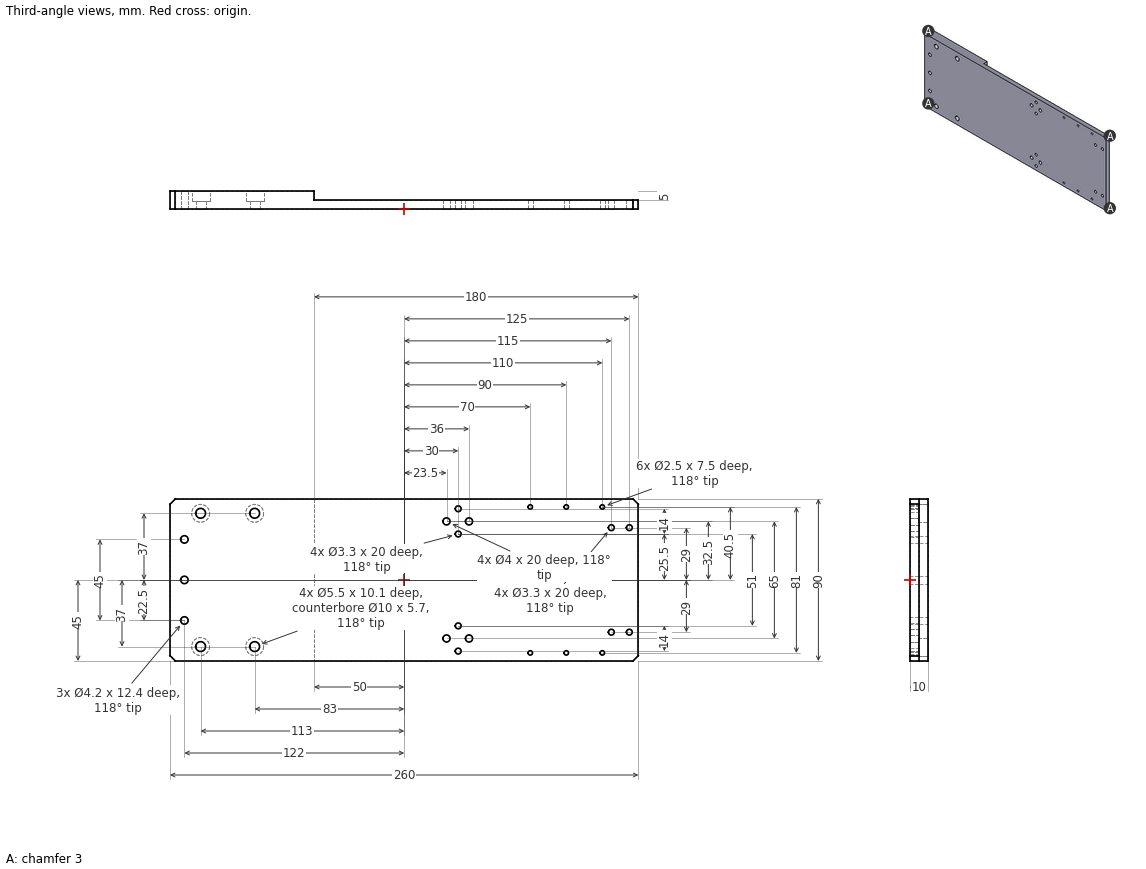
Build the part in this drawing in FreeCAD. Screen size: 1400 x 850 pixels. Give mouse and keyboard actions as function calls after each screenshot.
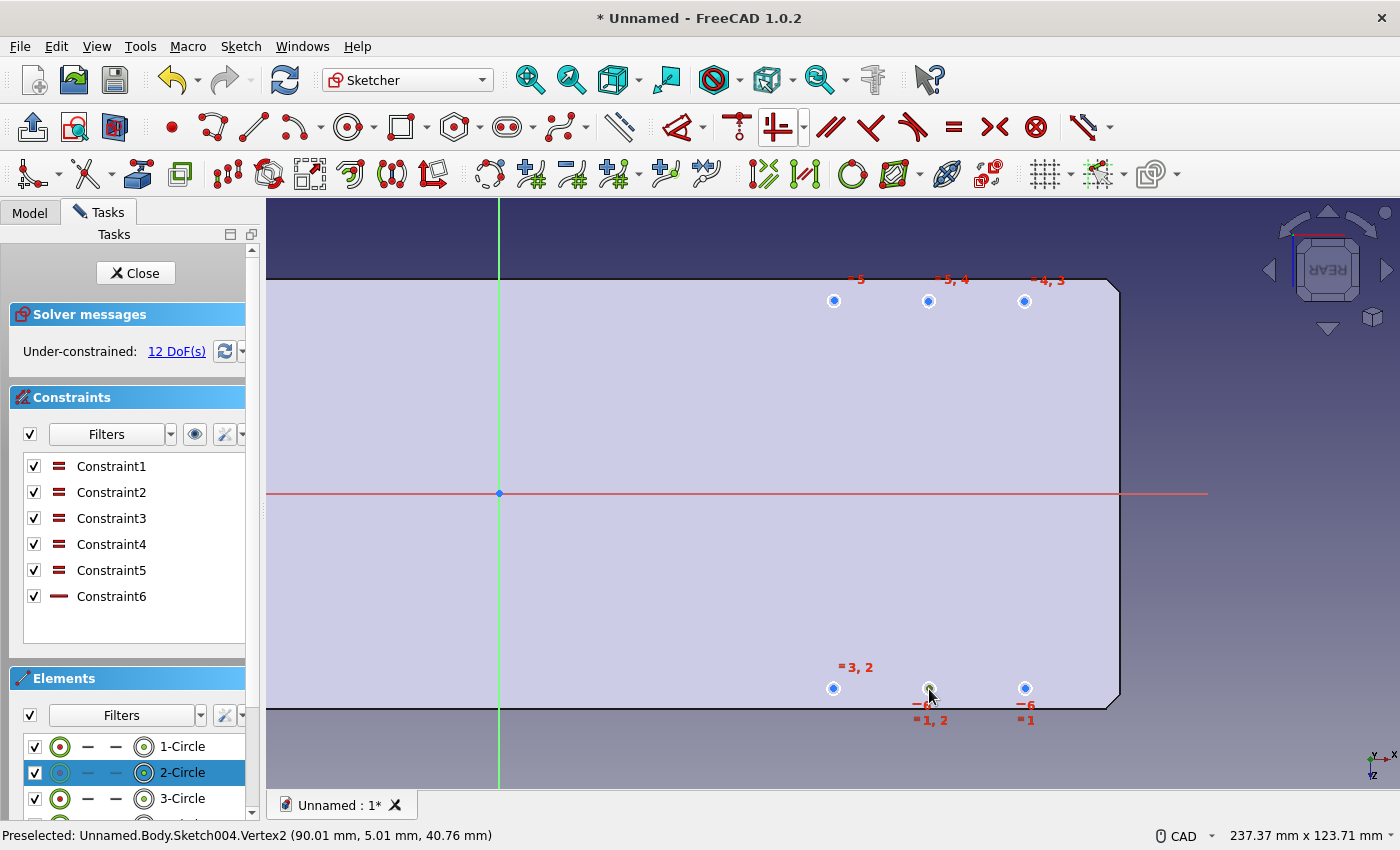
click(834, 689)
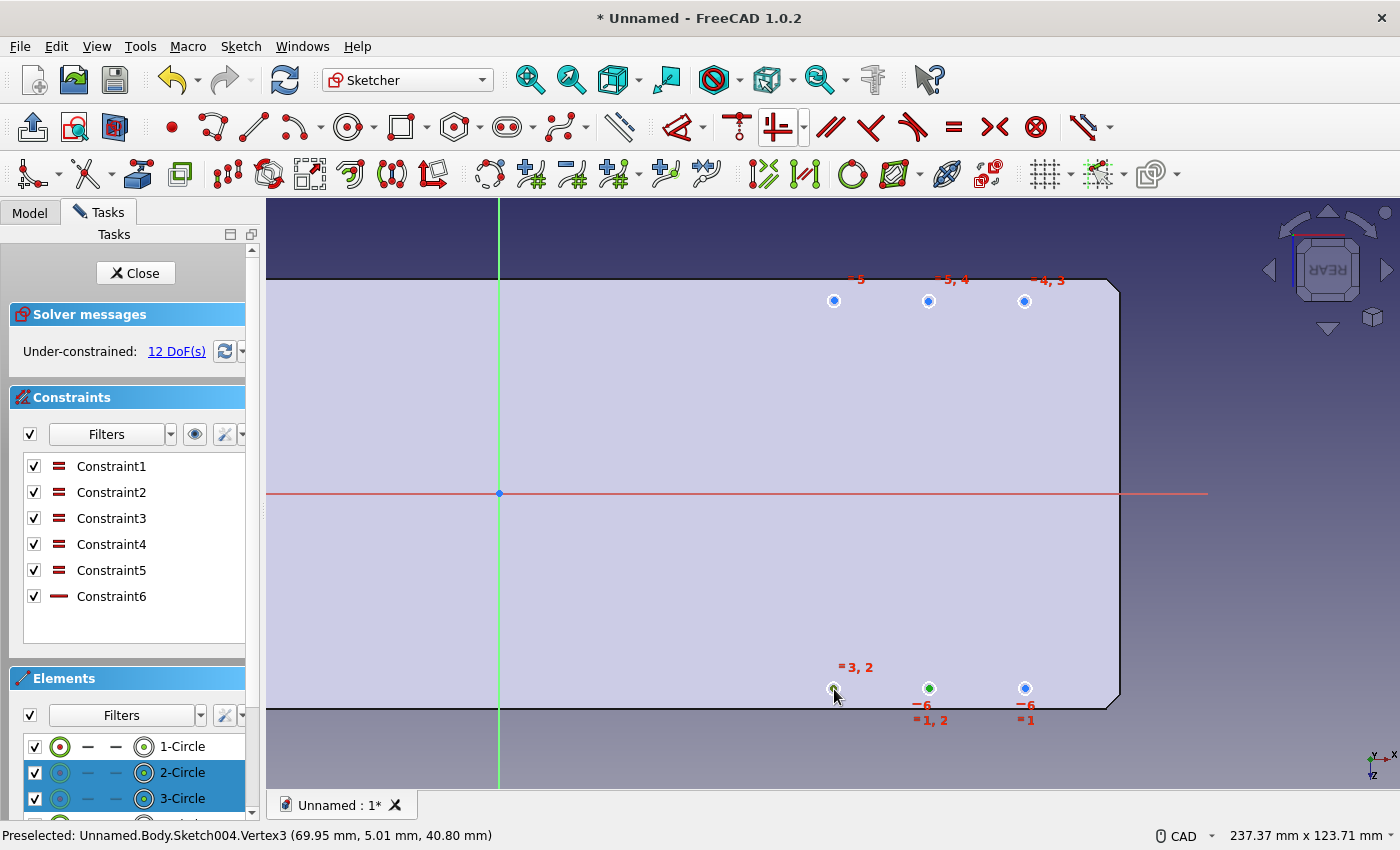
key(h)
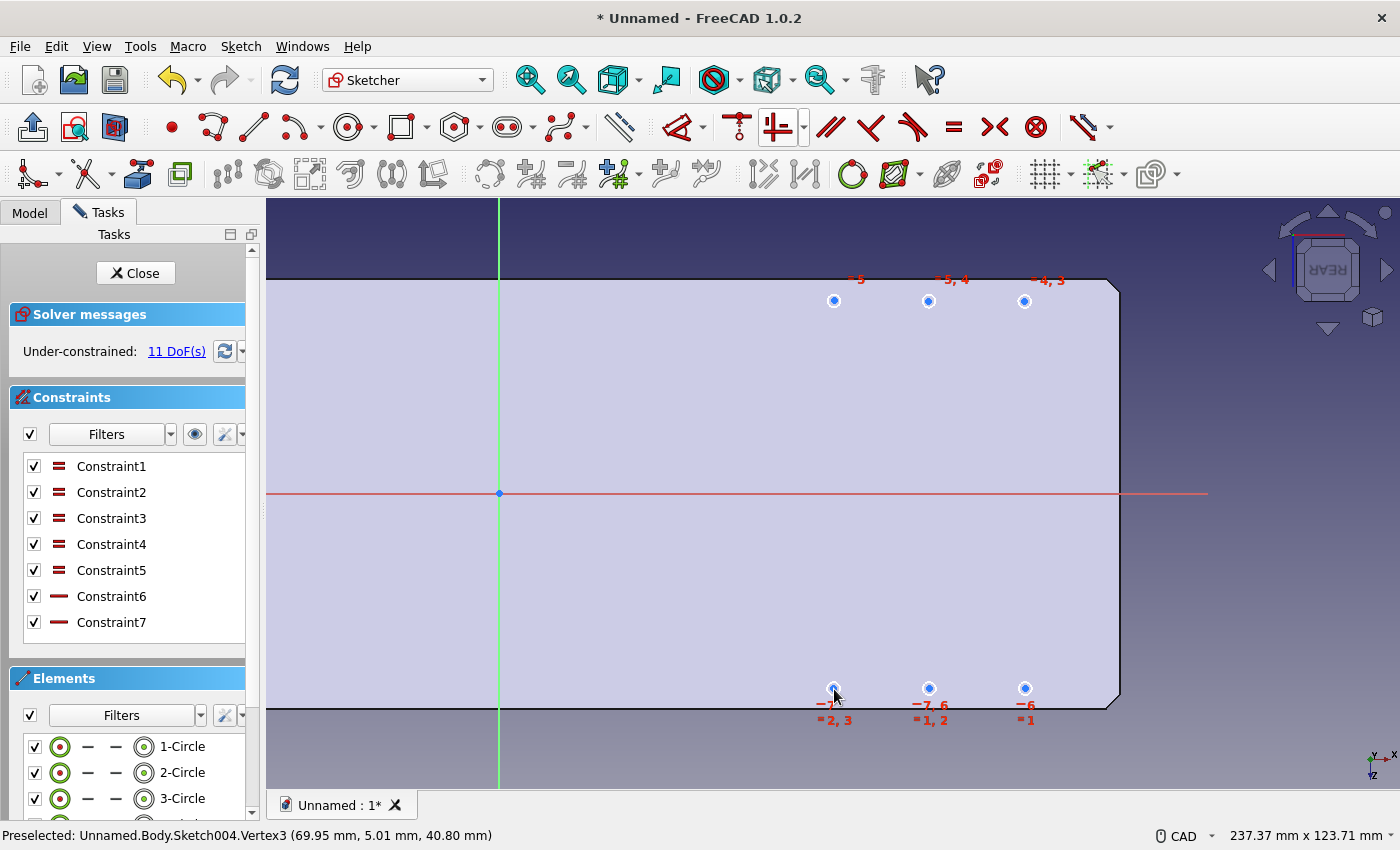
click(1025, 689)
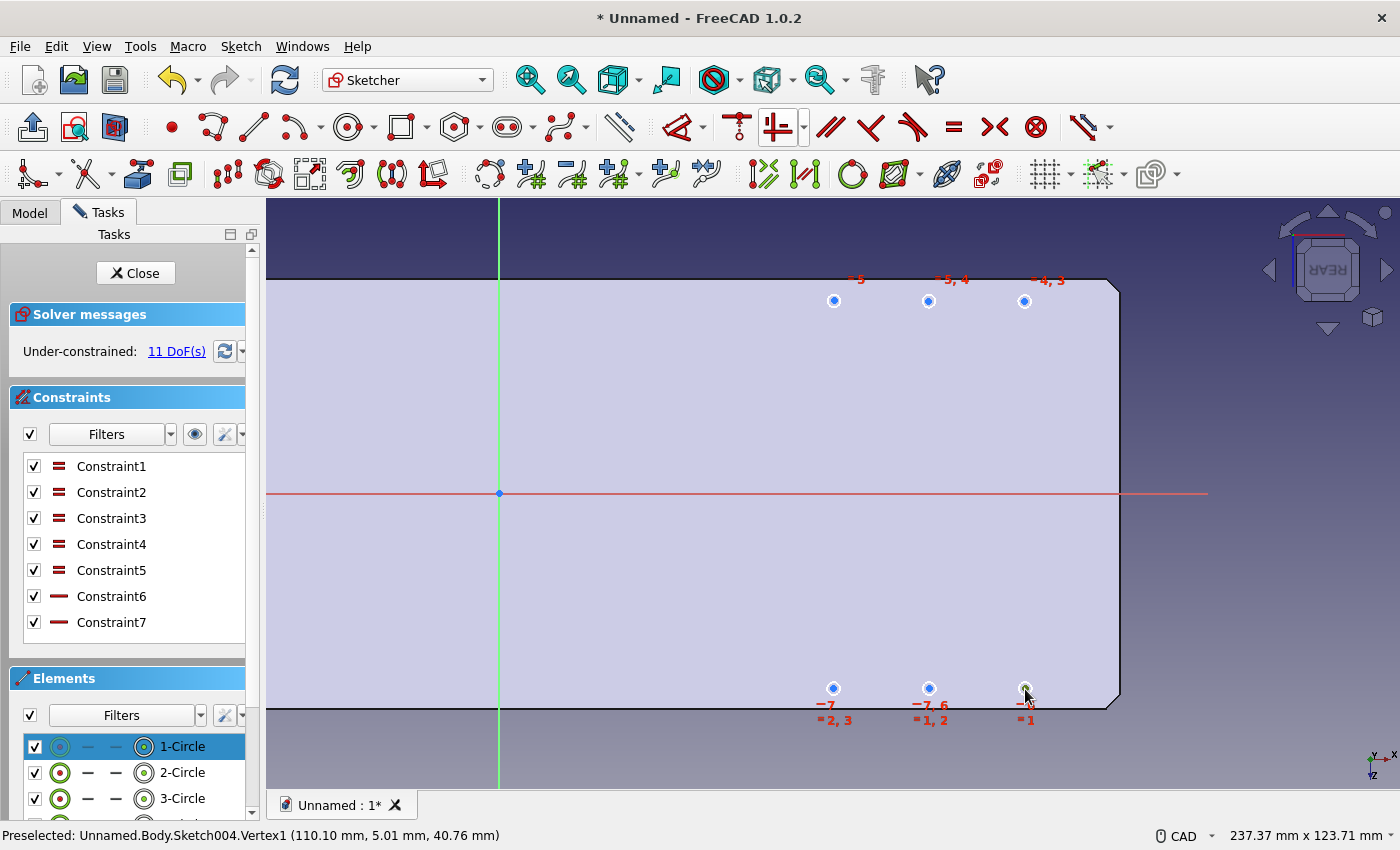
click(1025, 301)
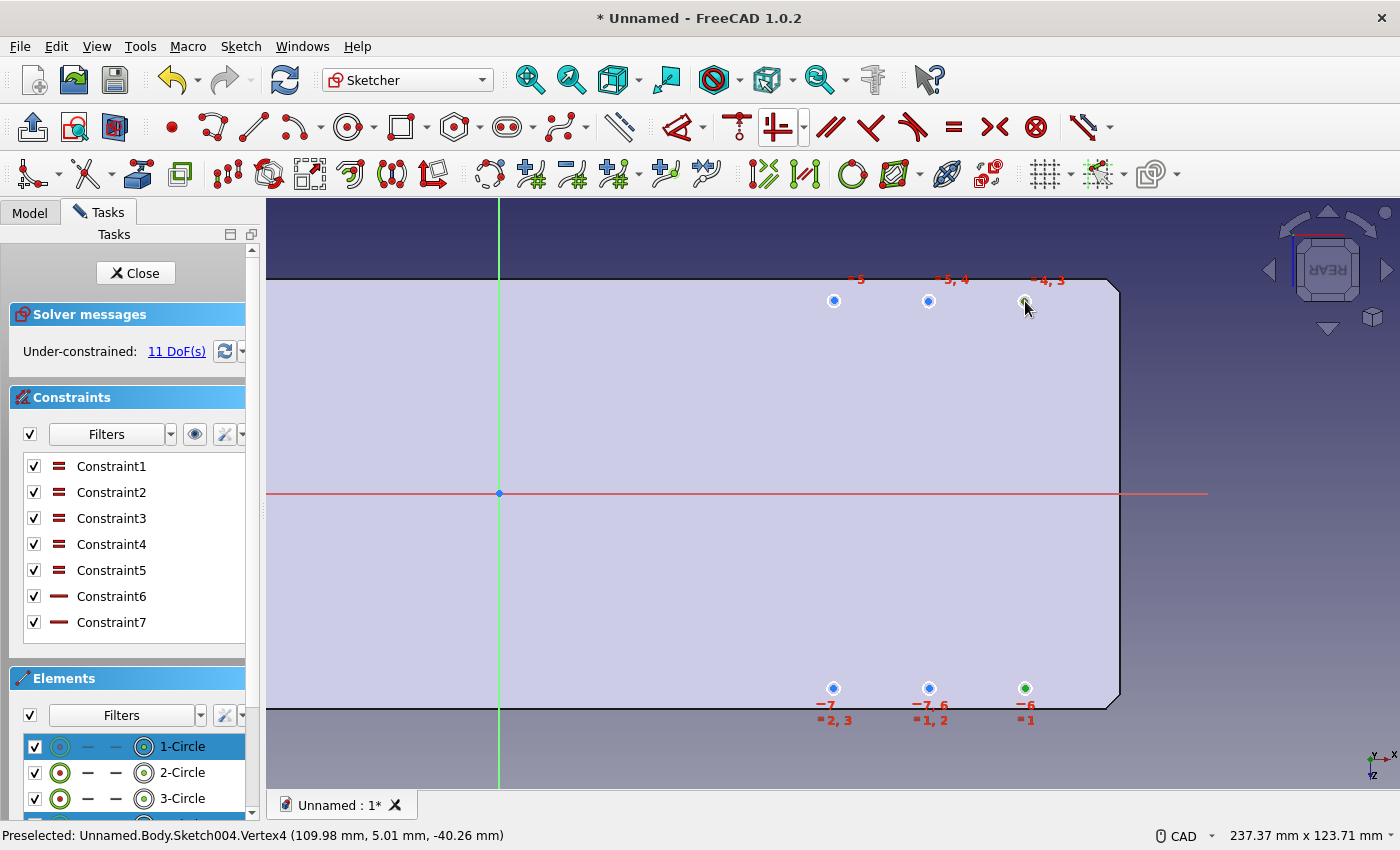
key(v)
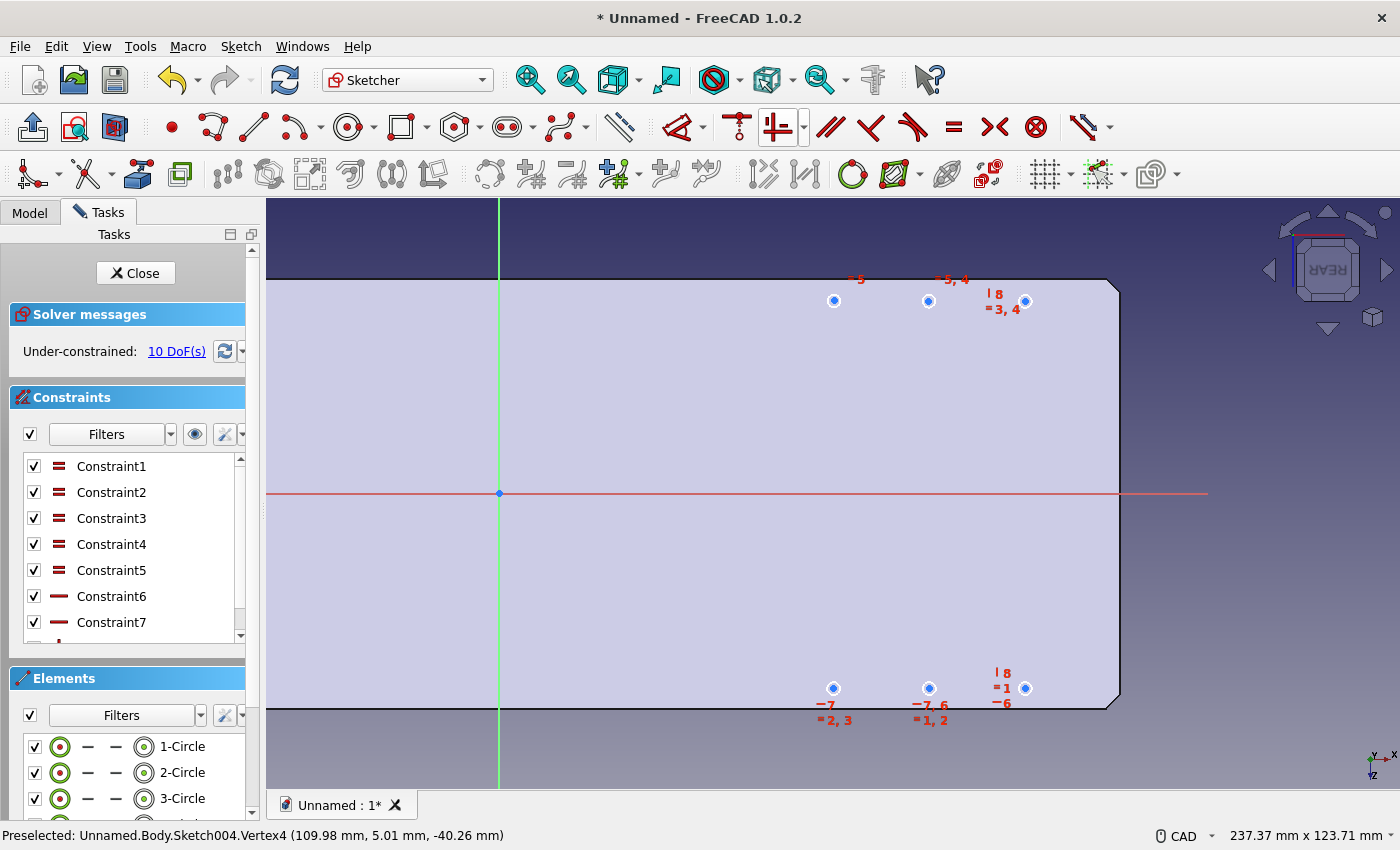
click(929, 689)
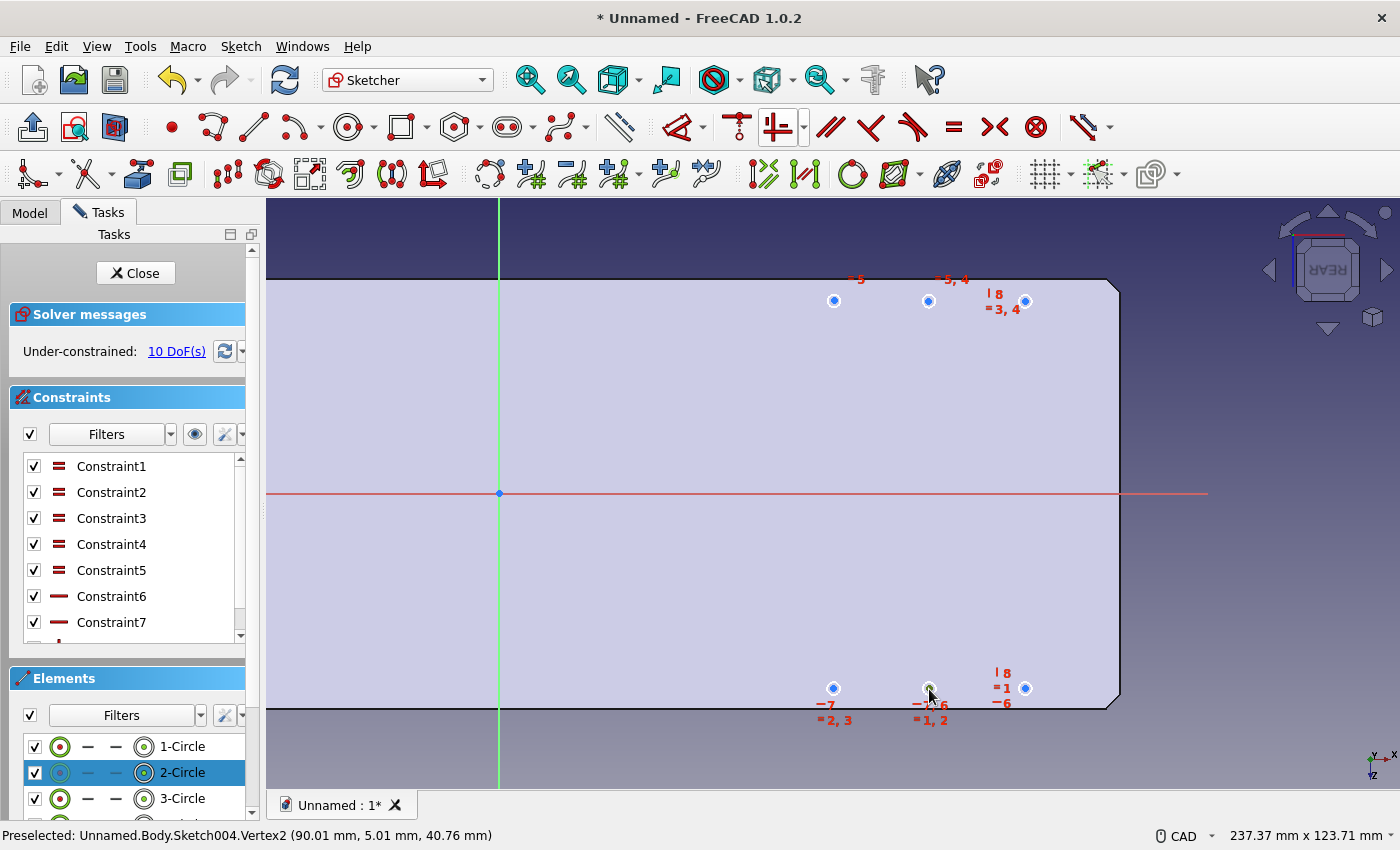
click(929, 301)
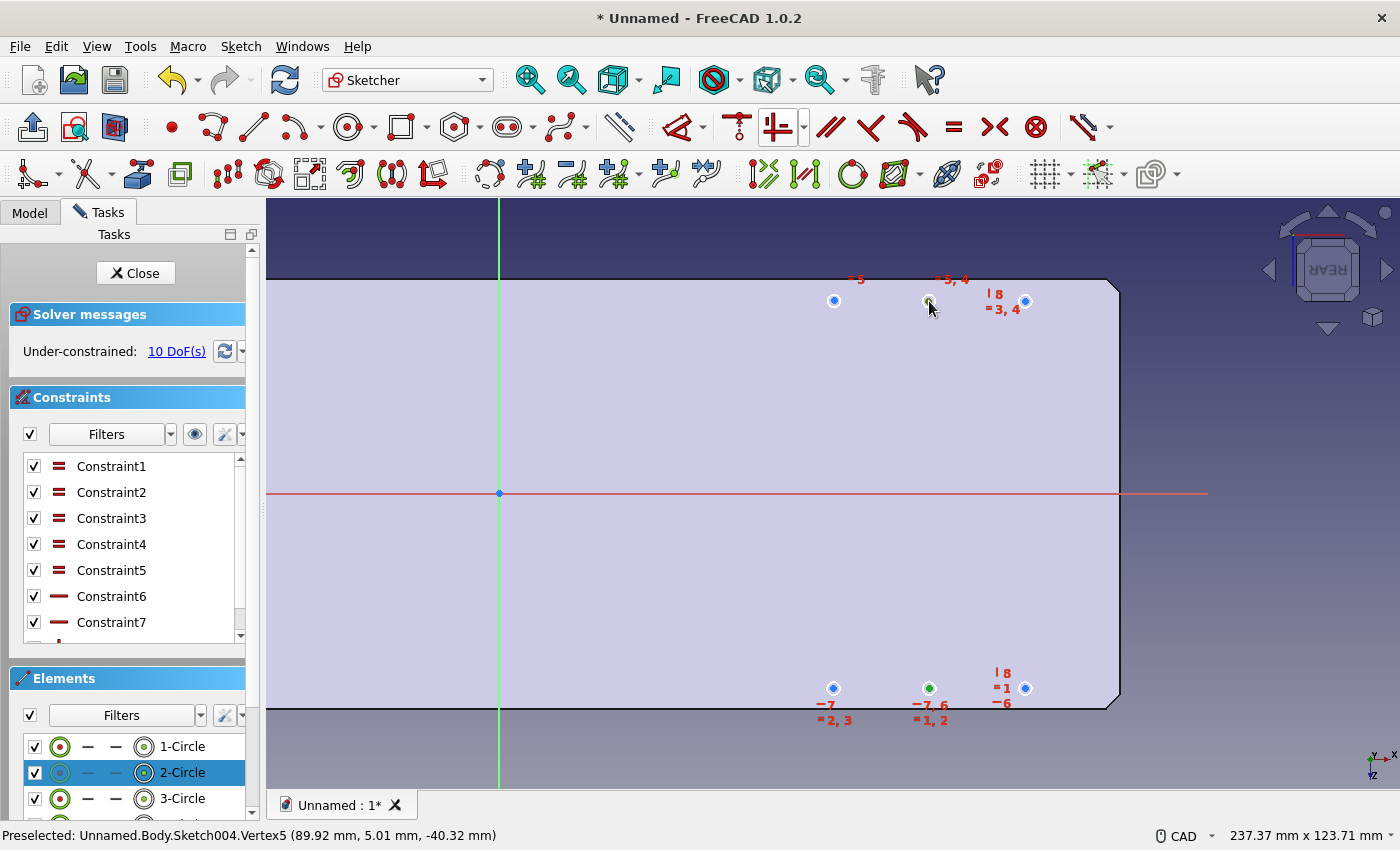
key(v)